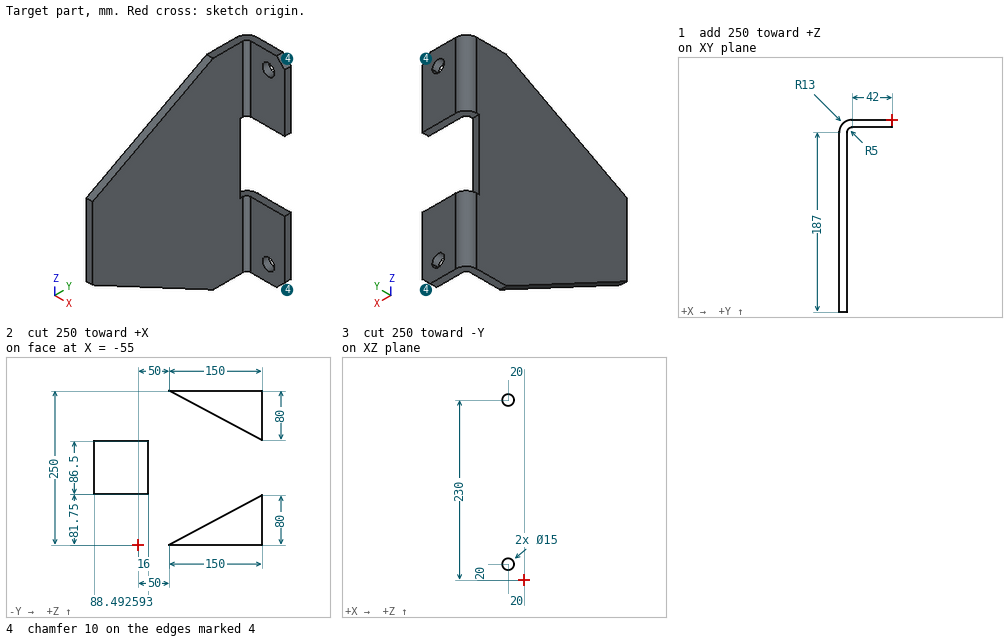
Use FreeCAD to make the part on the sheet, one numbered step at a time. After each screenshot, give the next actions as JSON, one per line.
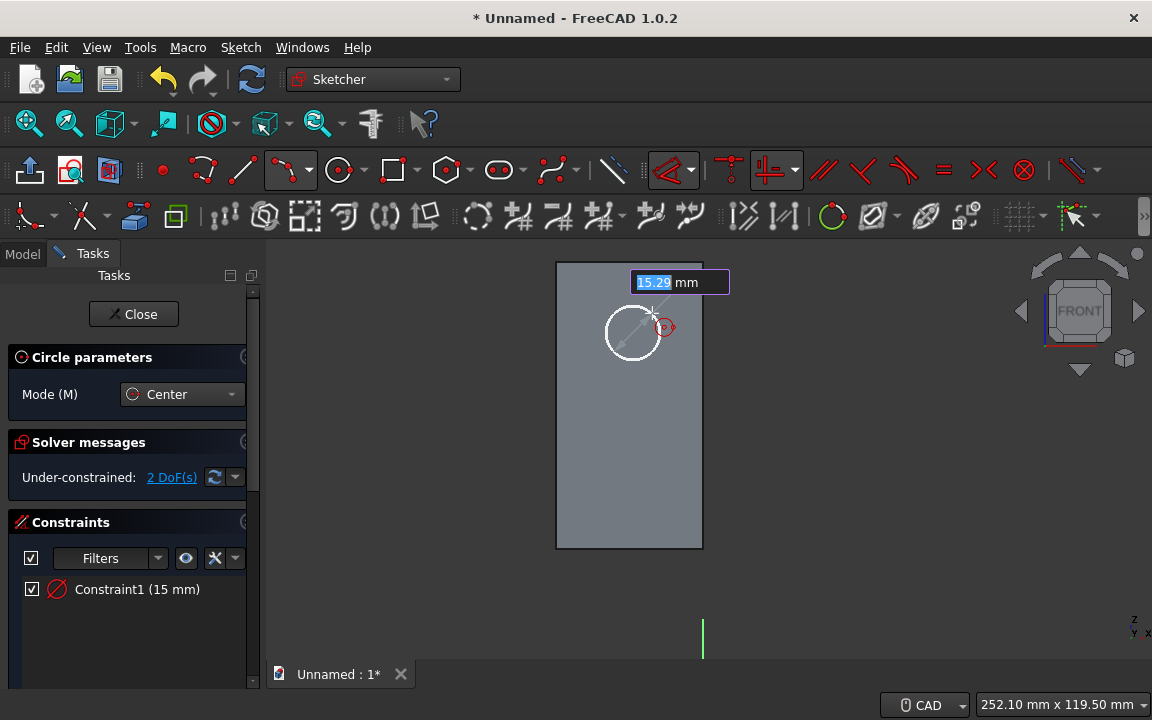
{"action": "type", "text": "15"}
{"action": "key", "text": "Return"}
{"action": "key", "text": "Escape"}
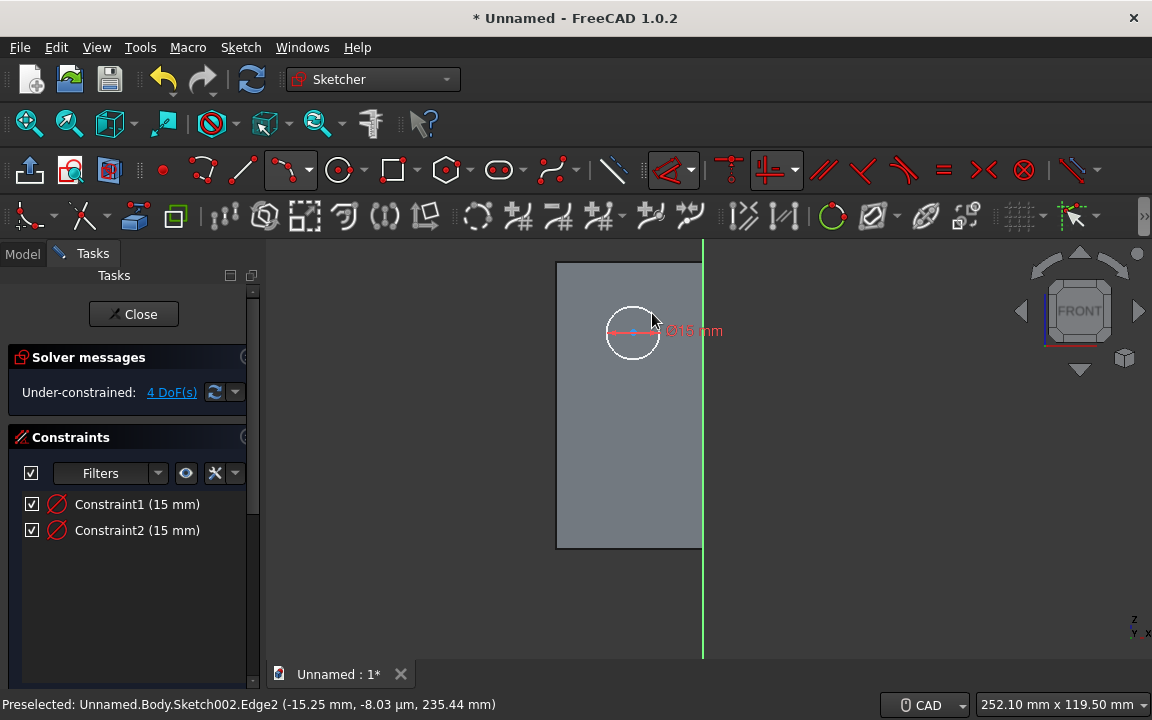
{"action": "scroll", "coordinate": [634, 331], "scroll_direction": "down", "scroll_amount": 6}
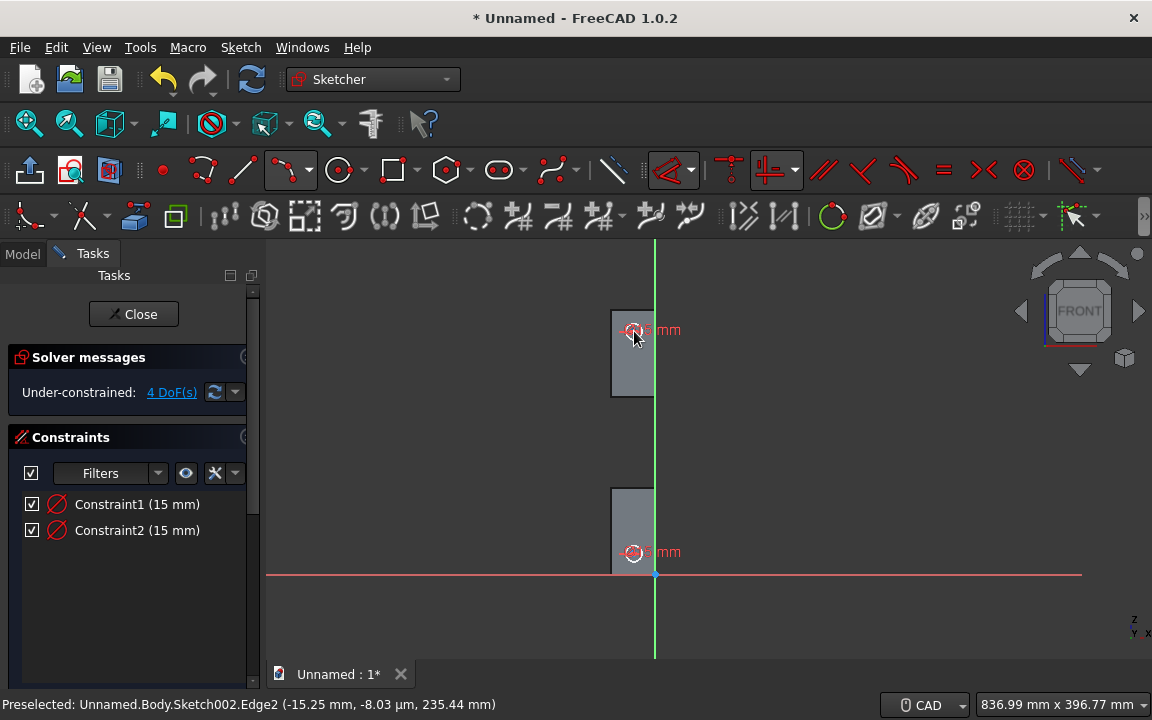
{"action": "scroll", "coordinate": [634, 554], "scroll_direction": "up", "scroll_amount": 4}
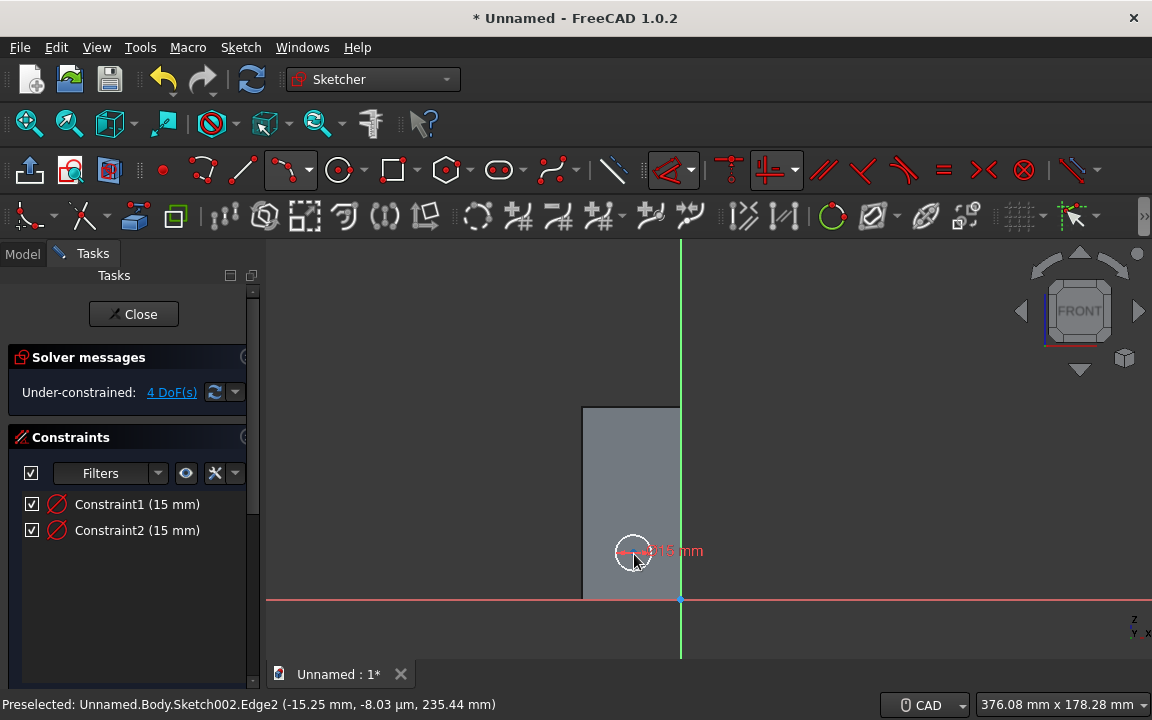
{"action": "left_click", "coordinate": [633, 553]}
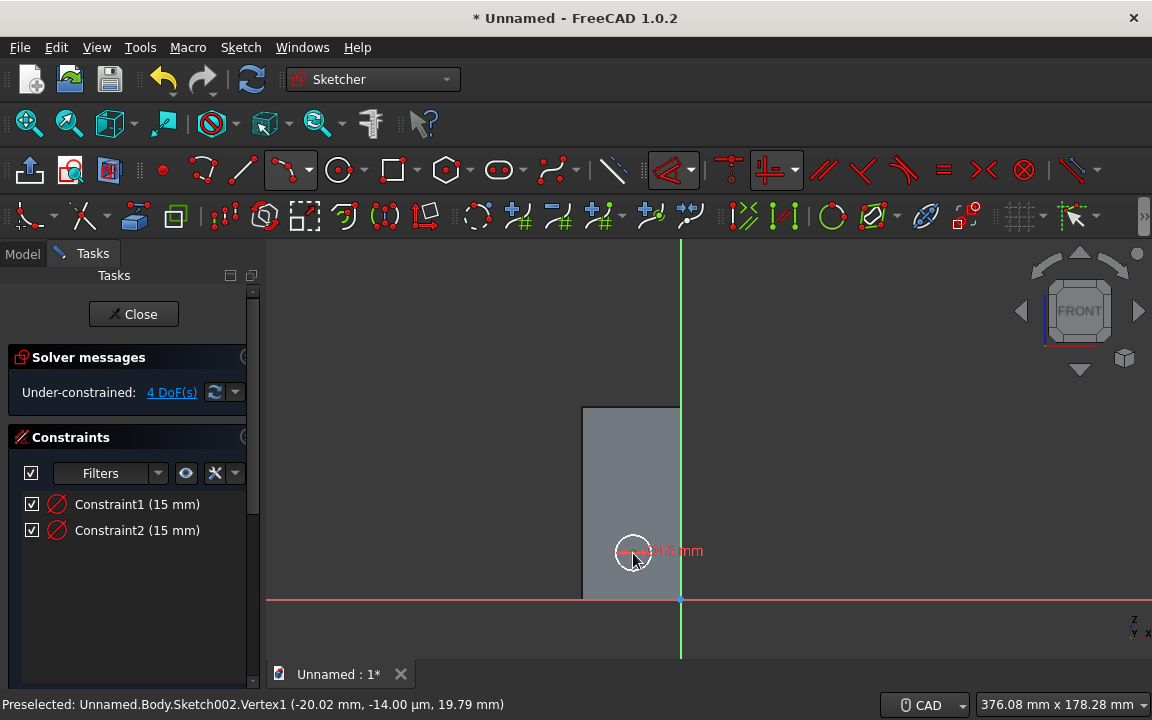
{"action": "left_click", "coordinate": [694, 170]}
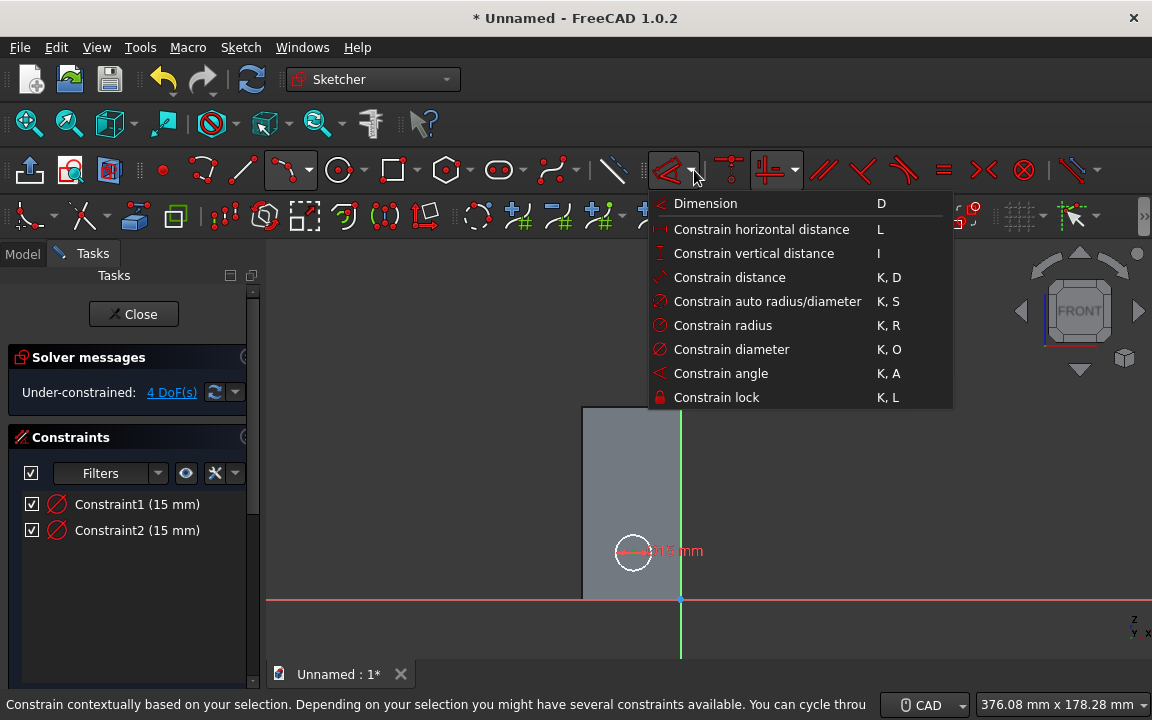
{"action": "left_click", "coordinate": [801, 229]}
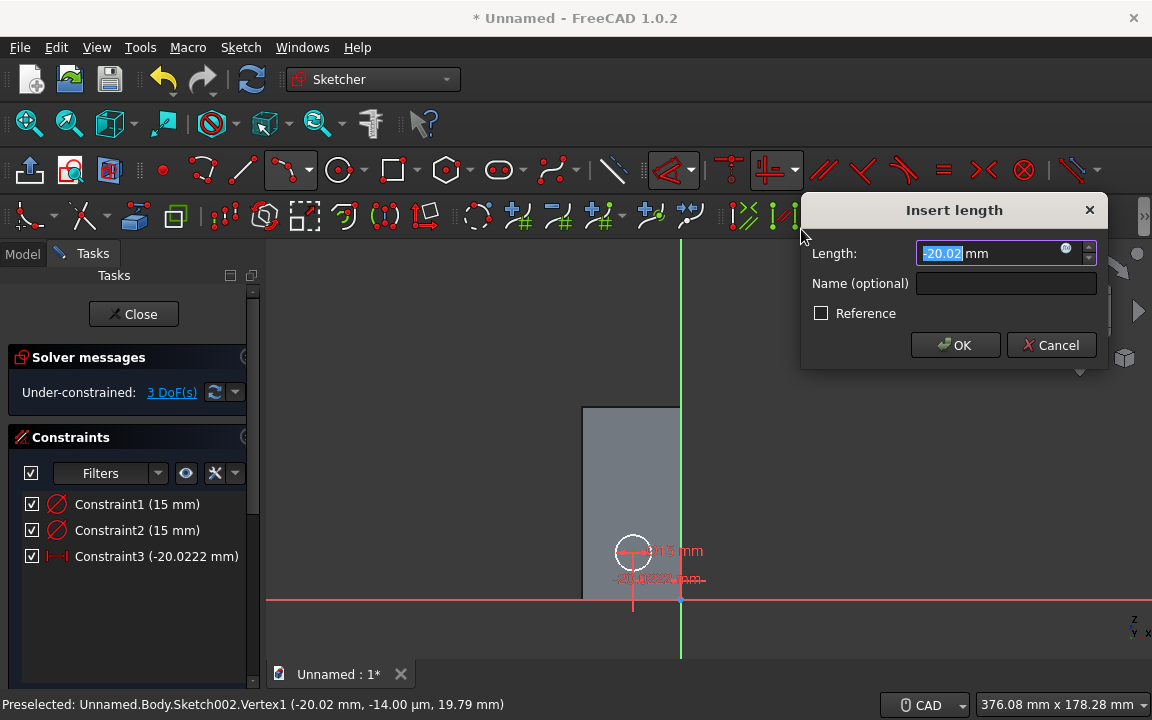
{"action": "type", "text": "-20"}
{"action": "key", "text": "Return"}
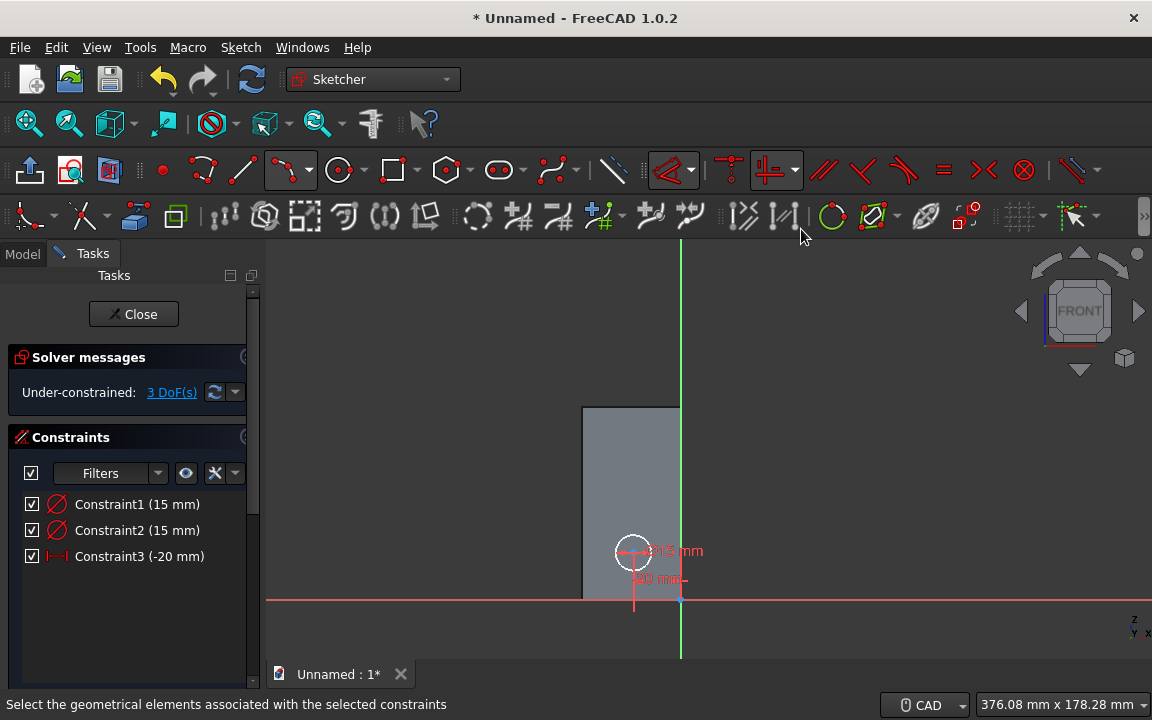
{"action": "left_click", "coordinate": [634, 553]}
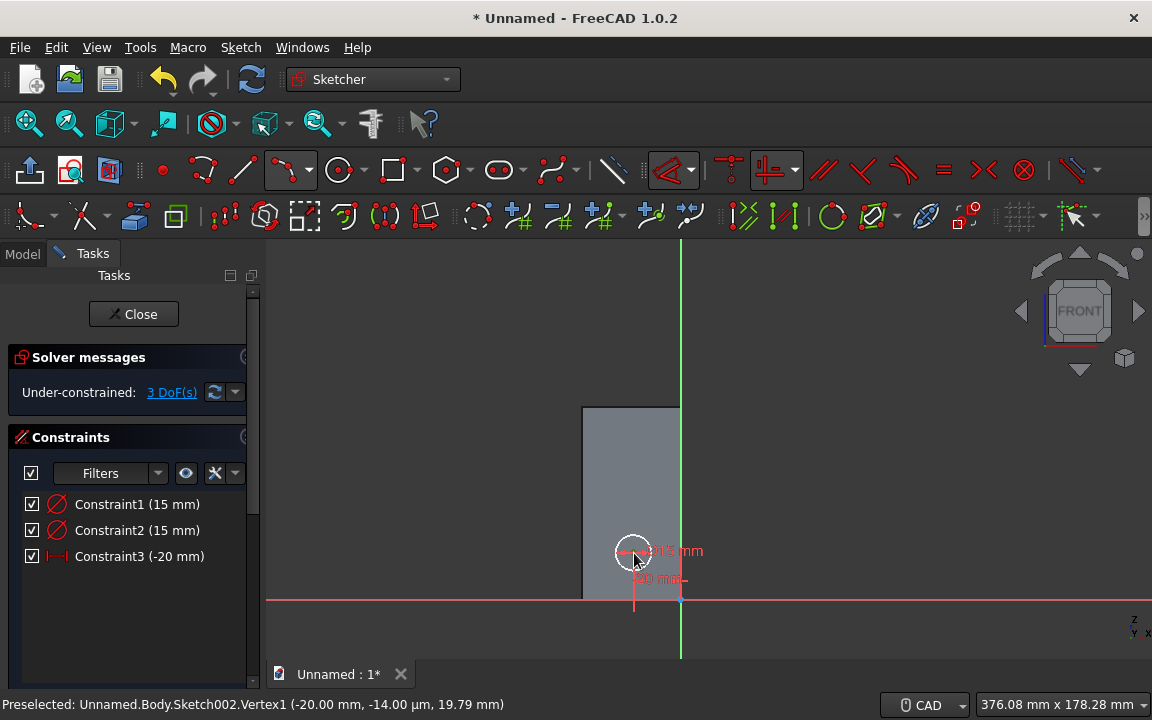
{"action": "key", "text": "i"}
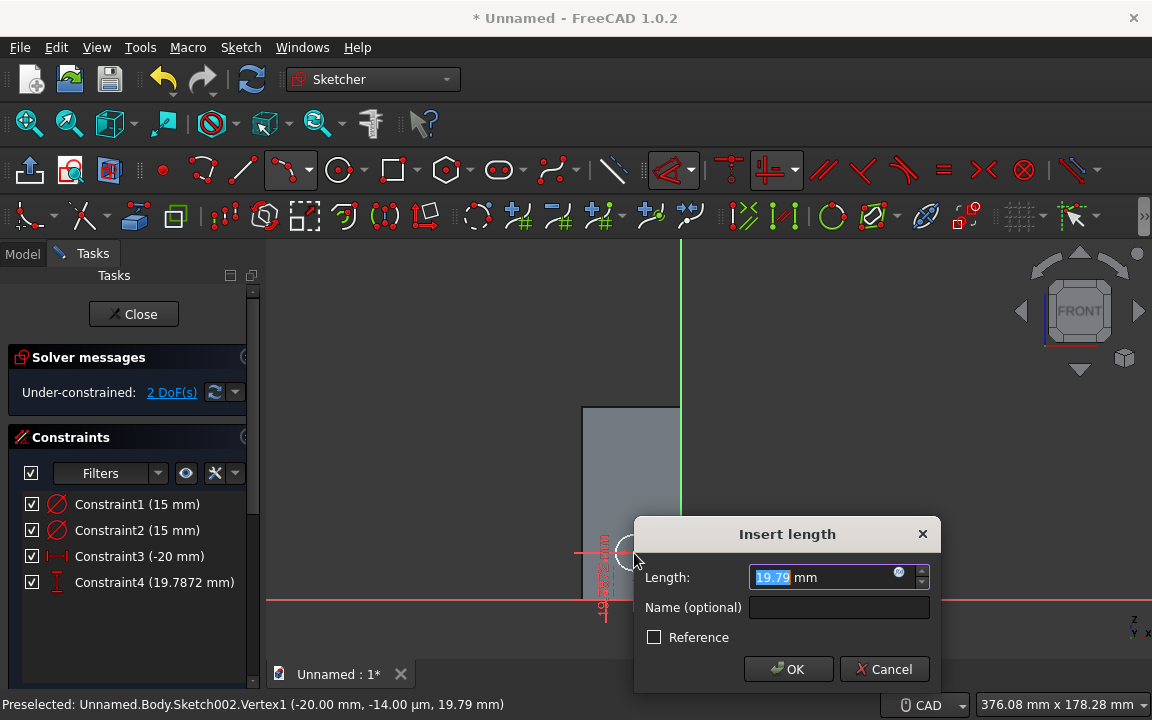
{"action": "type", "text": "20"}
{"action": "key", "text": "Return"}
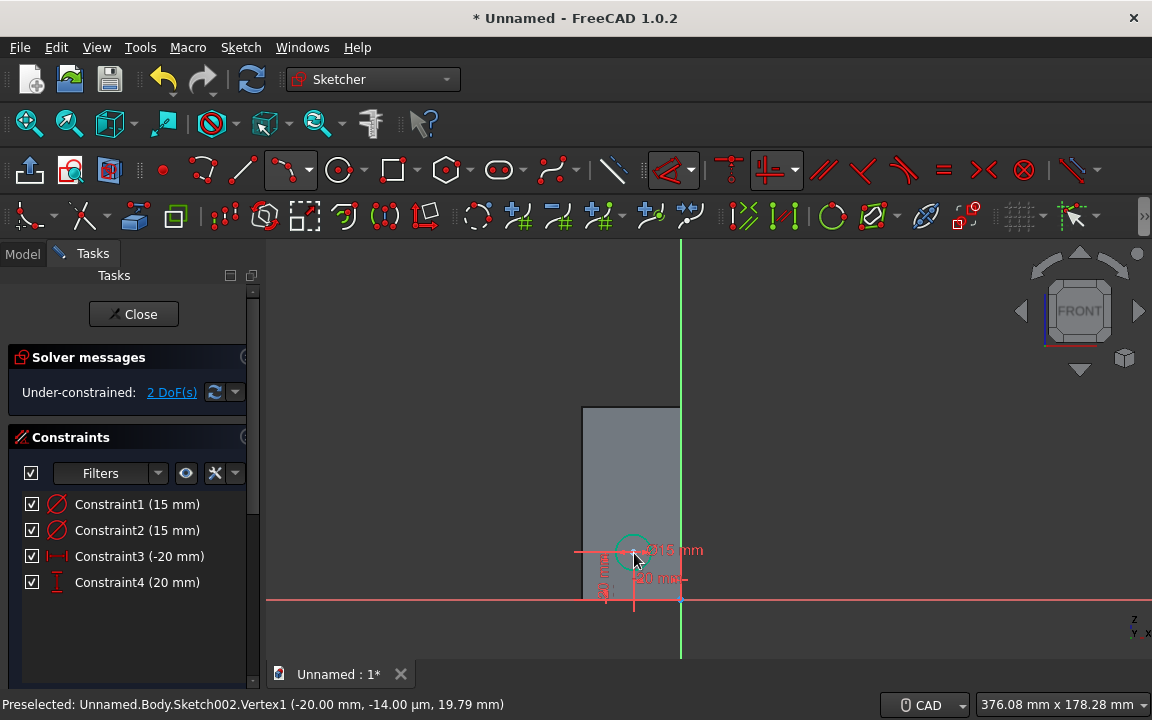
{"action": "scroll", "coordinate": [634, 554], "scroll_direction": "down", "scroll_amount": 4}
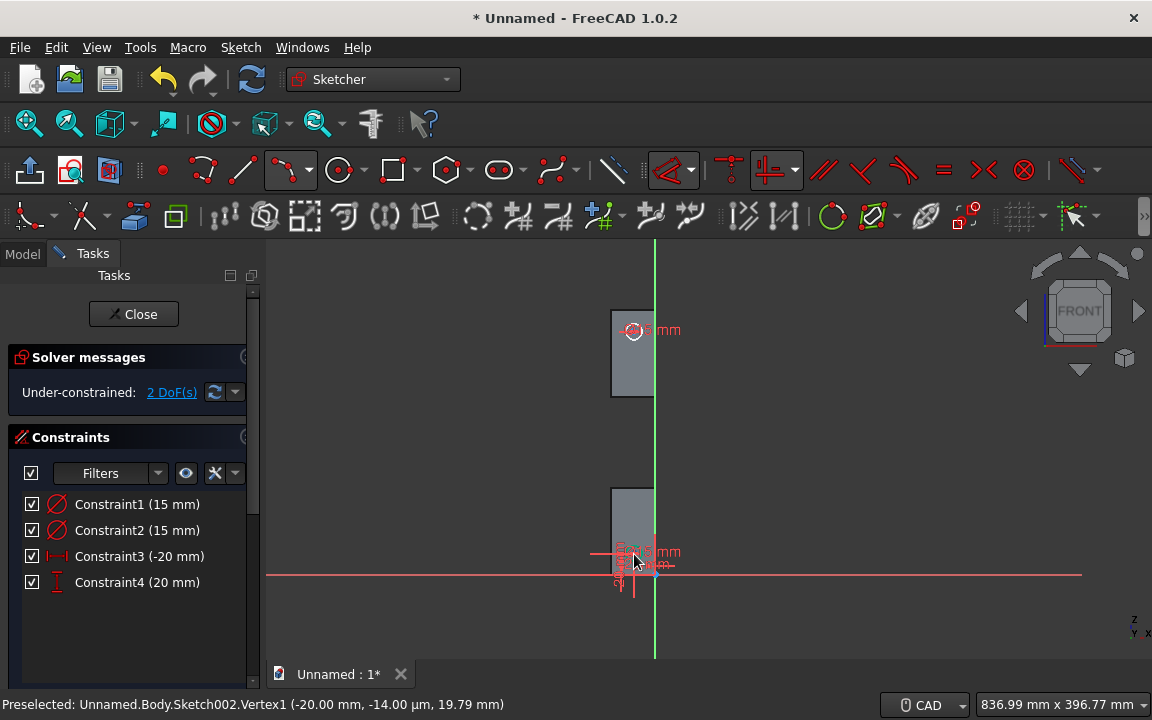
{"action": "scroll", "coordinate": [634, 332], "scroll_direction": "up", "scroll_amount": 4}